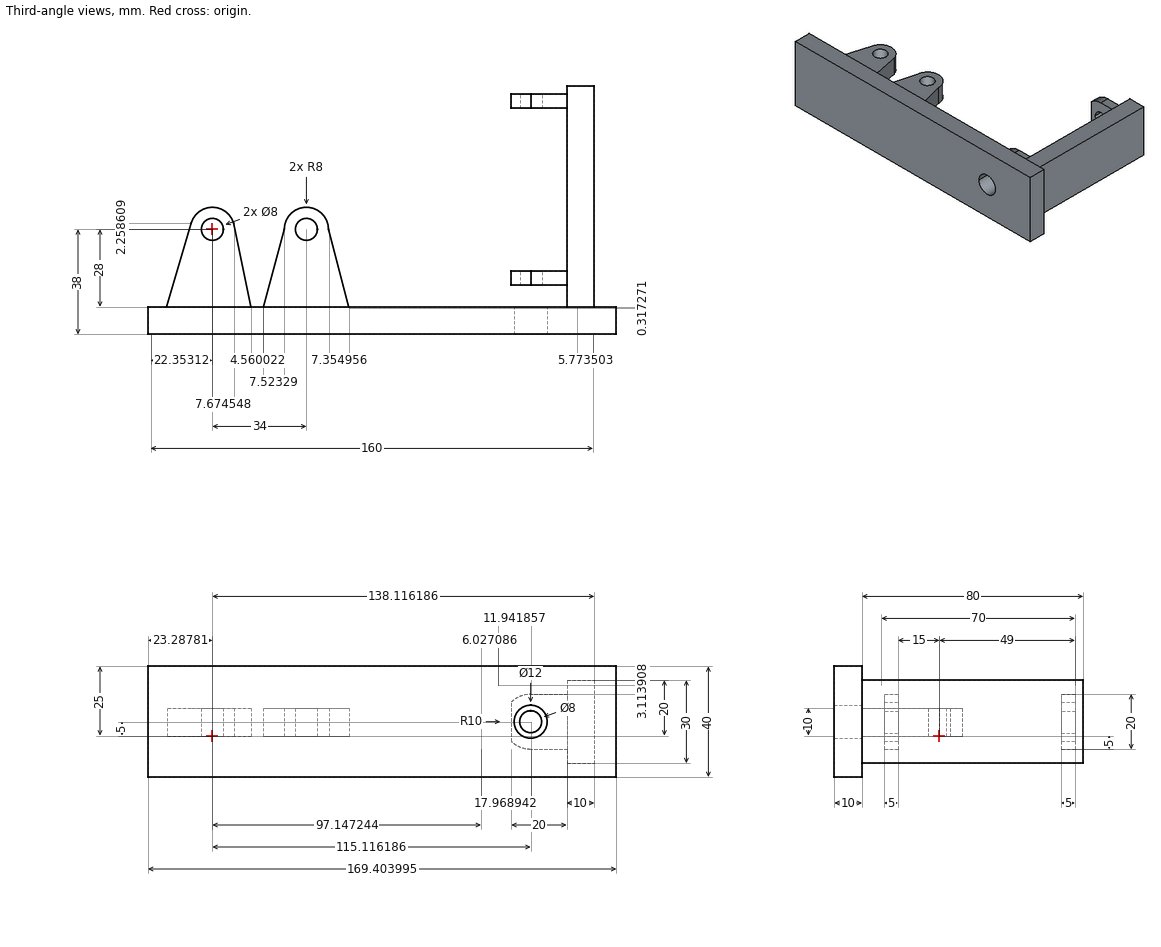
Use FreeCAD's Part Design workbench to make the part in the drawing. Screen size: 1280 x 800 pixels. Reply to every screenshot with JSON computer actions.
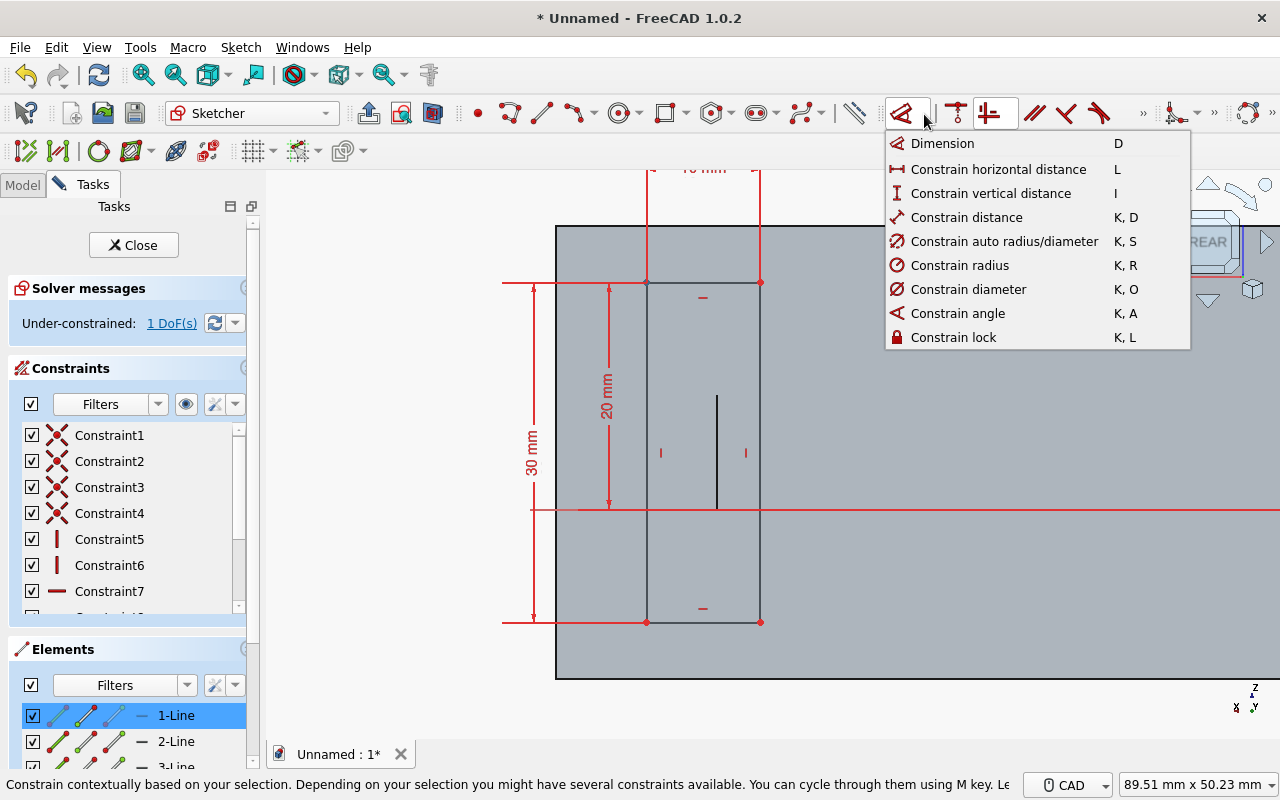
{"action": "left_click", "coordinate": [1038, 169]}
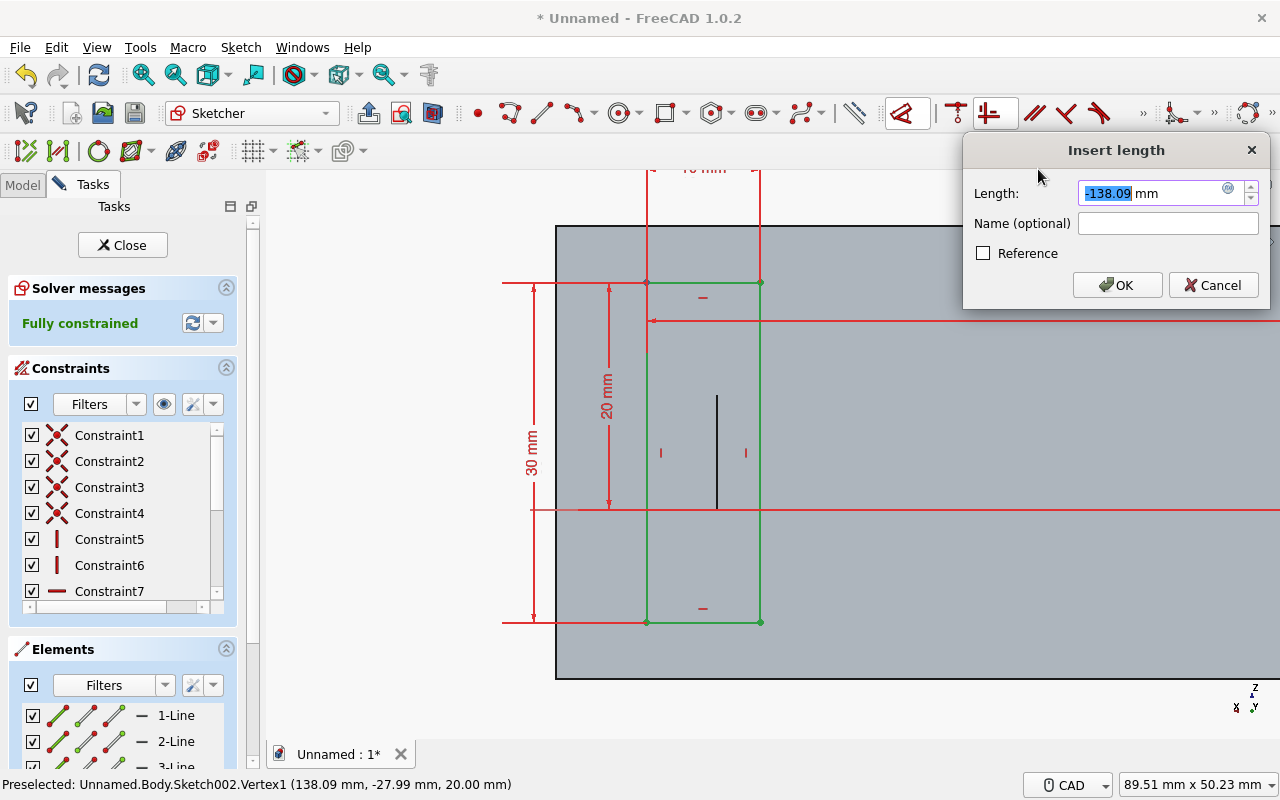
{"action": "type", "text": "-138.116186"}
{"action": "key", "text": "Return"}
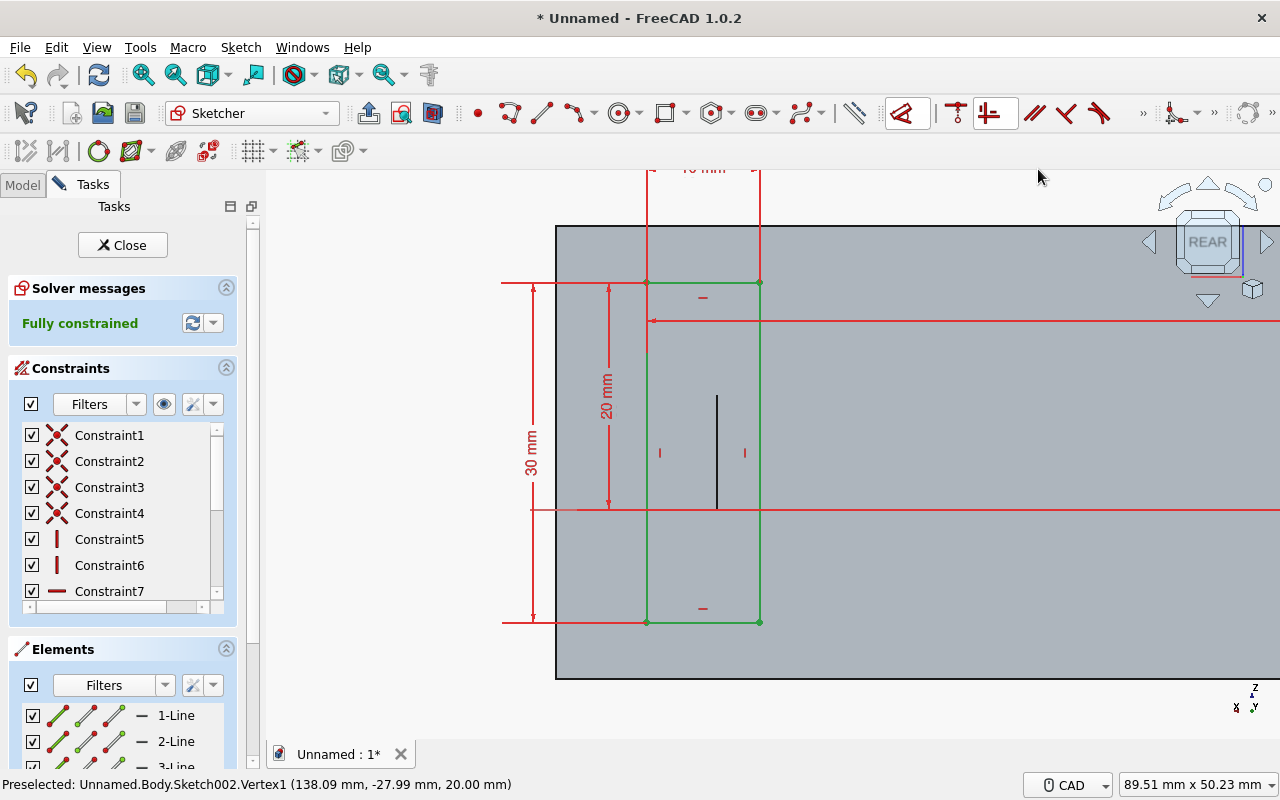
{"action": "left_click", "coordinate": [123, 245]}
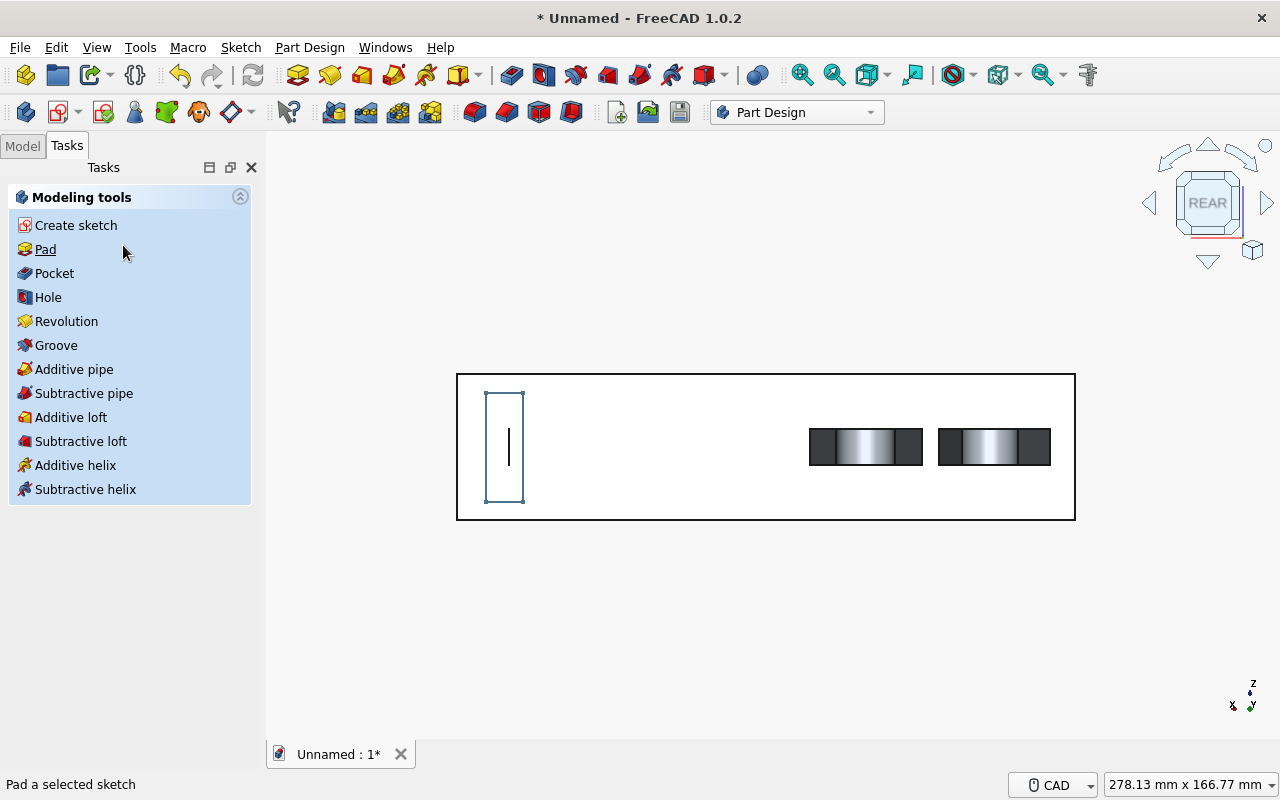
{"action": "left_click", "coordinate": [298, 76]}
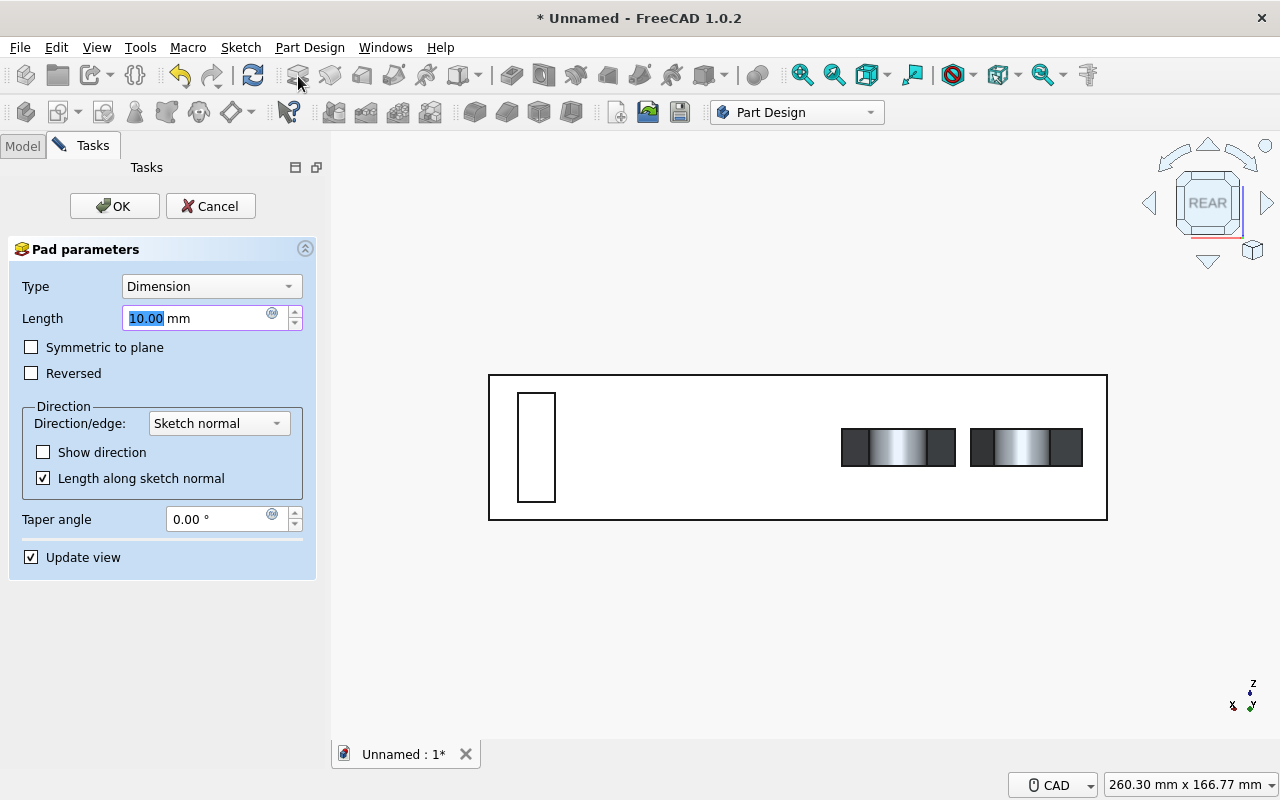
{"action": "type", "text": "80"}
{"action": "key", "text": "Tab"}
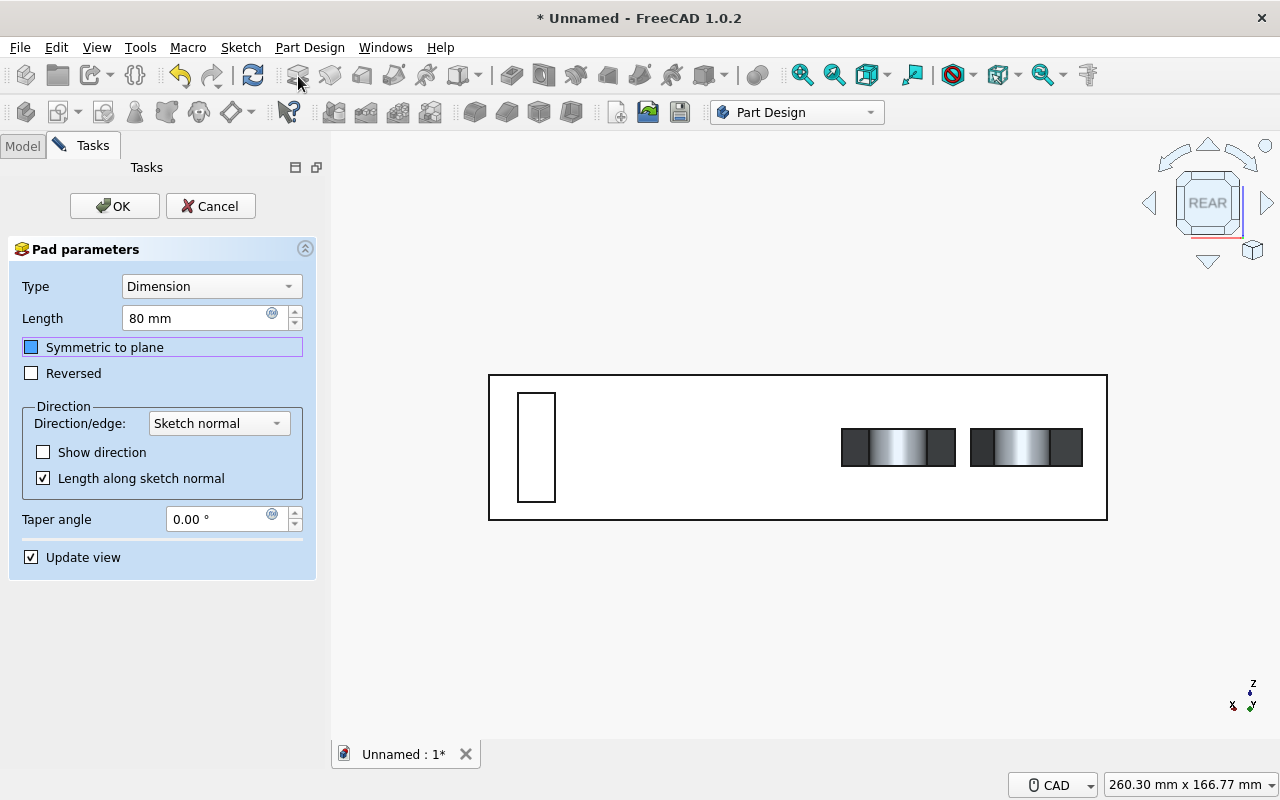
{"action": "left_click", "coordinate": [115, 206]}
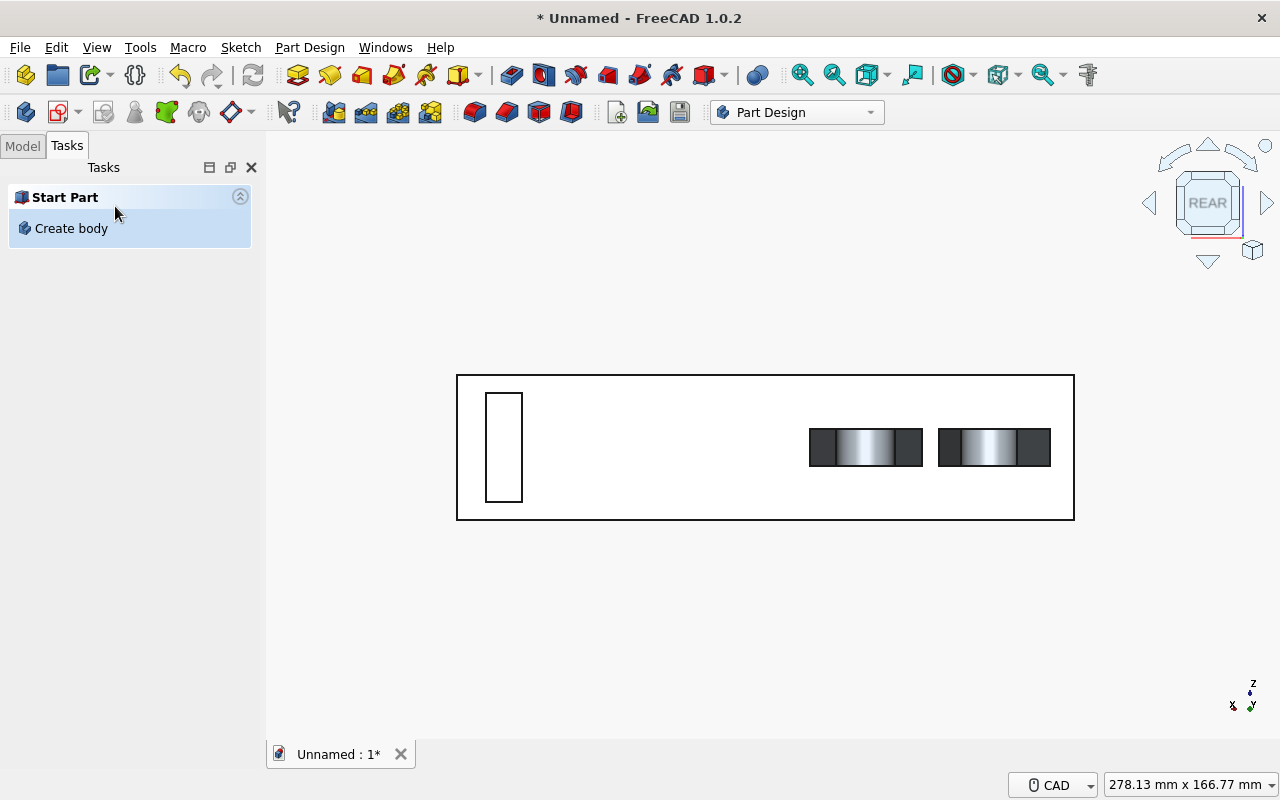
{"action": "key", "text": "6"}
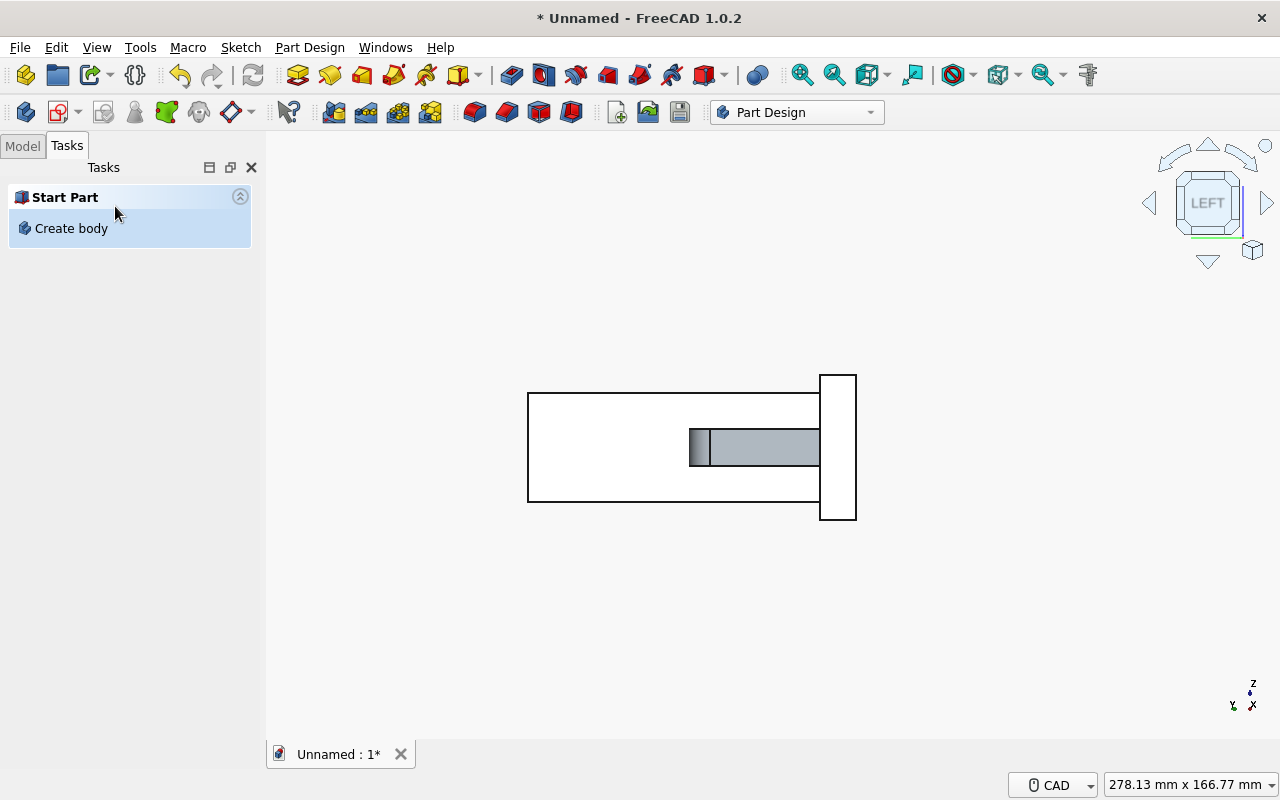
{"action": "left_click", "coordinate": [804, 76]}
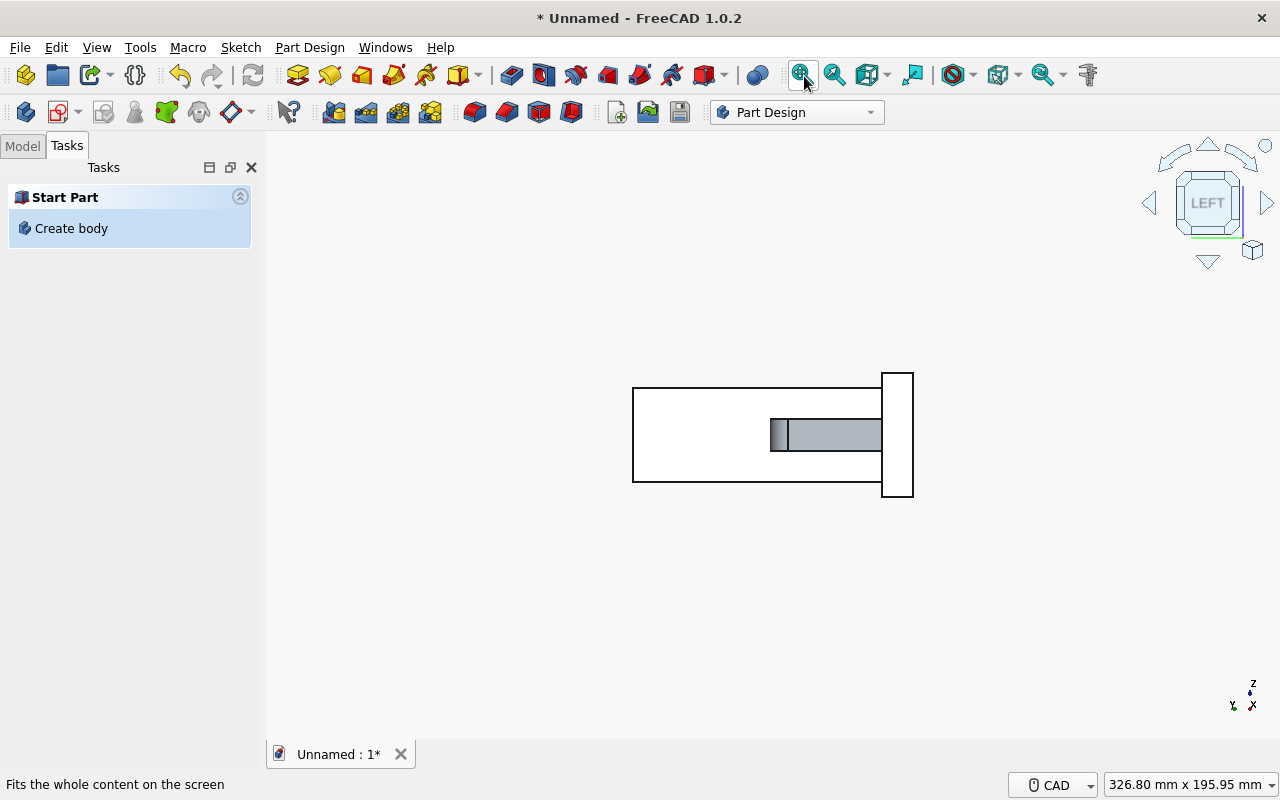
{"action": "left_click", "coordinate": [687, 434]}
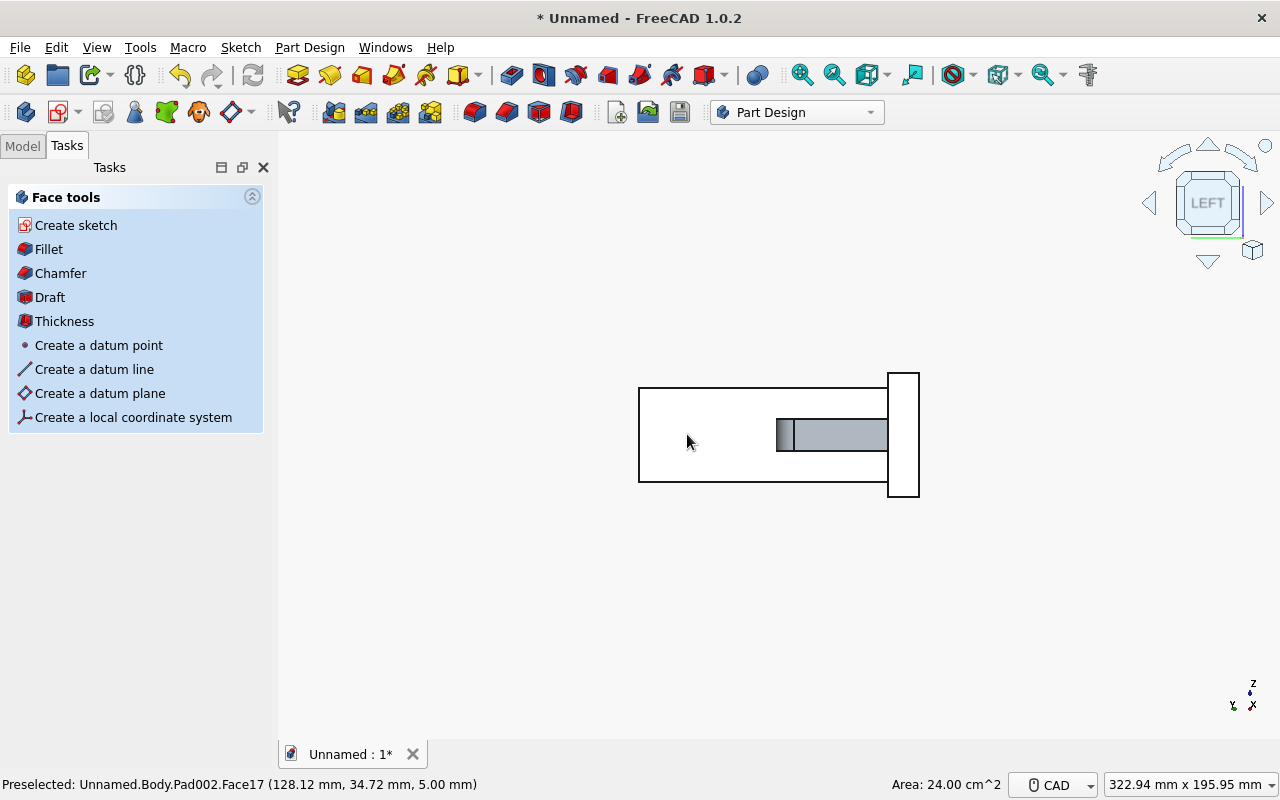
{"action": "left_click", "coordinate": [58, 112]}